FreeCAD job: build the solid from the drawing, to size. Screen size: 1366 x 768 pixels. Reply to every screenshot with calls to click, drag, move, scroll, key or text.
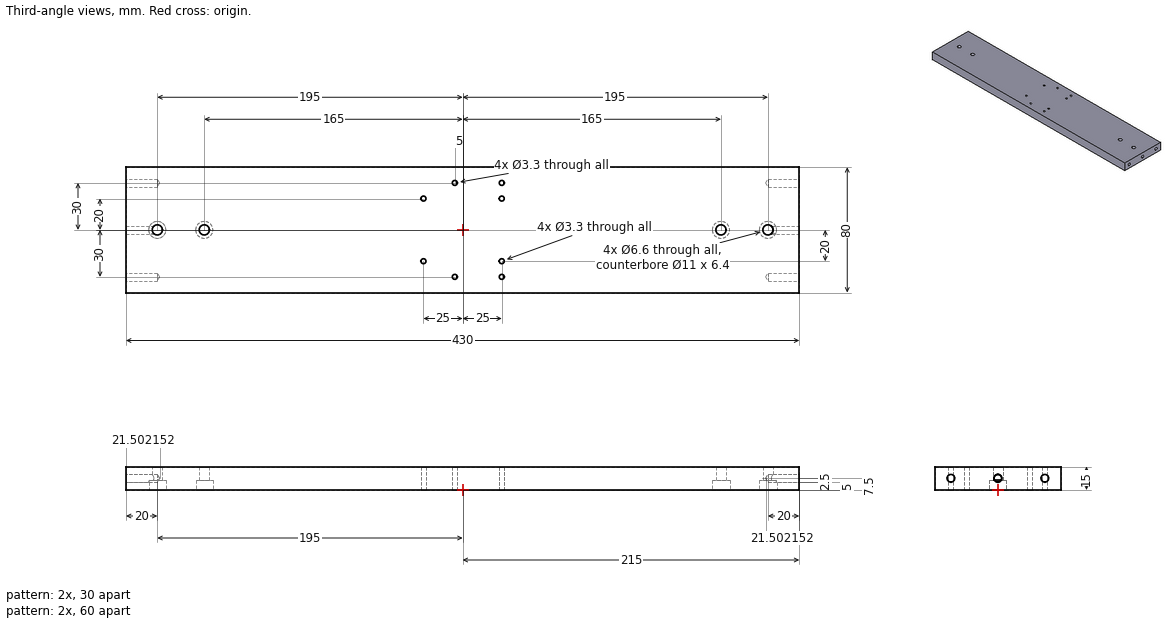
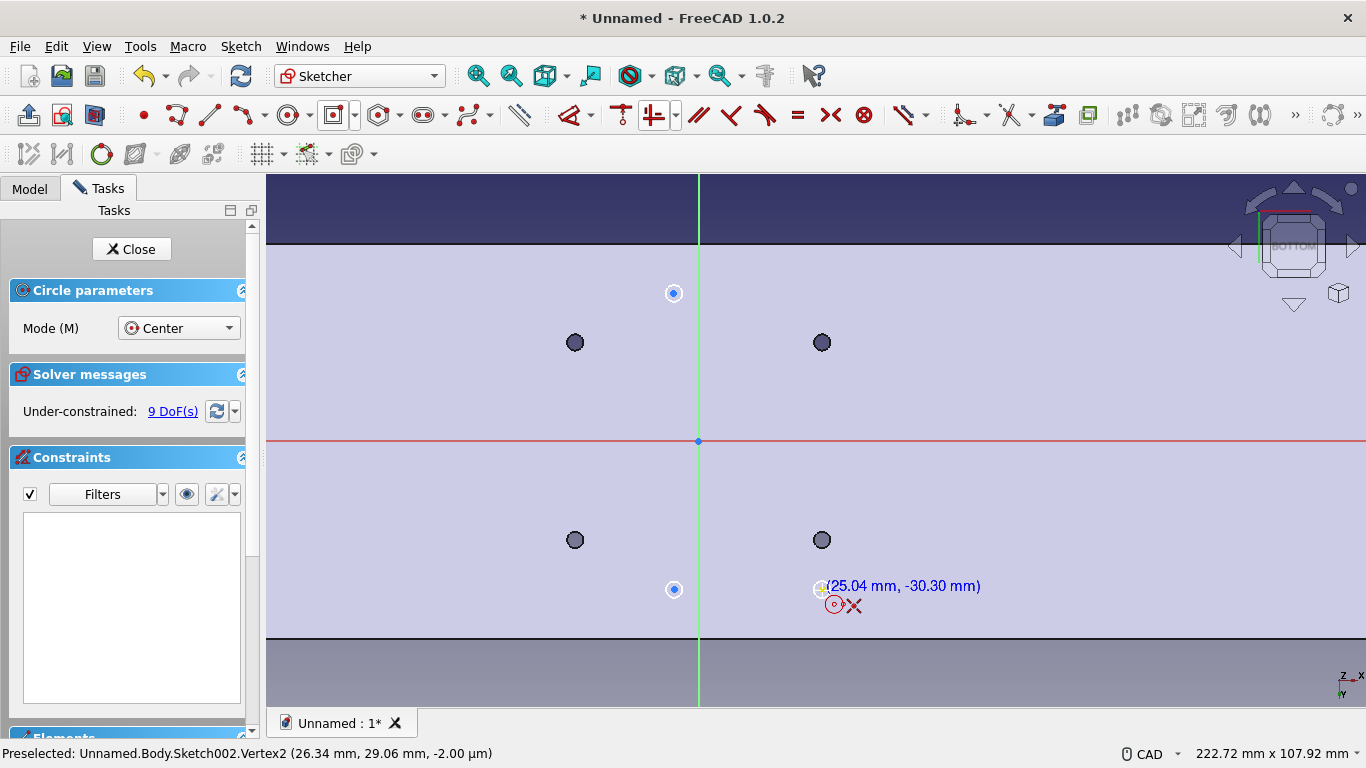
scroll(822, 293, up, 6)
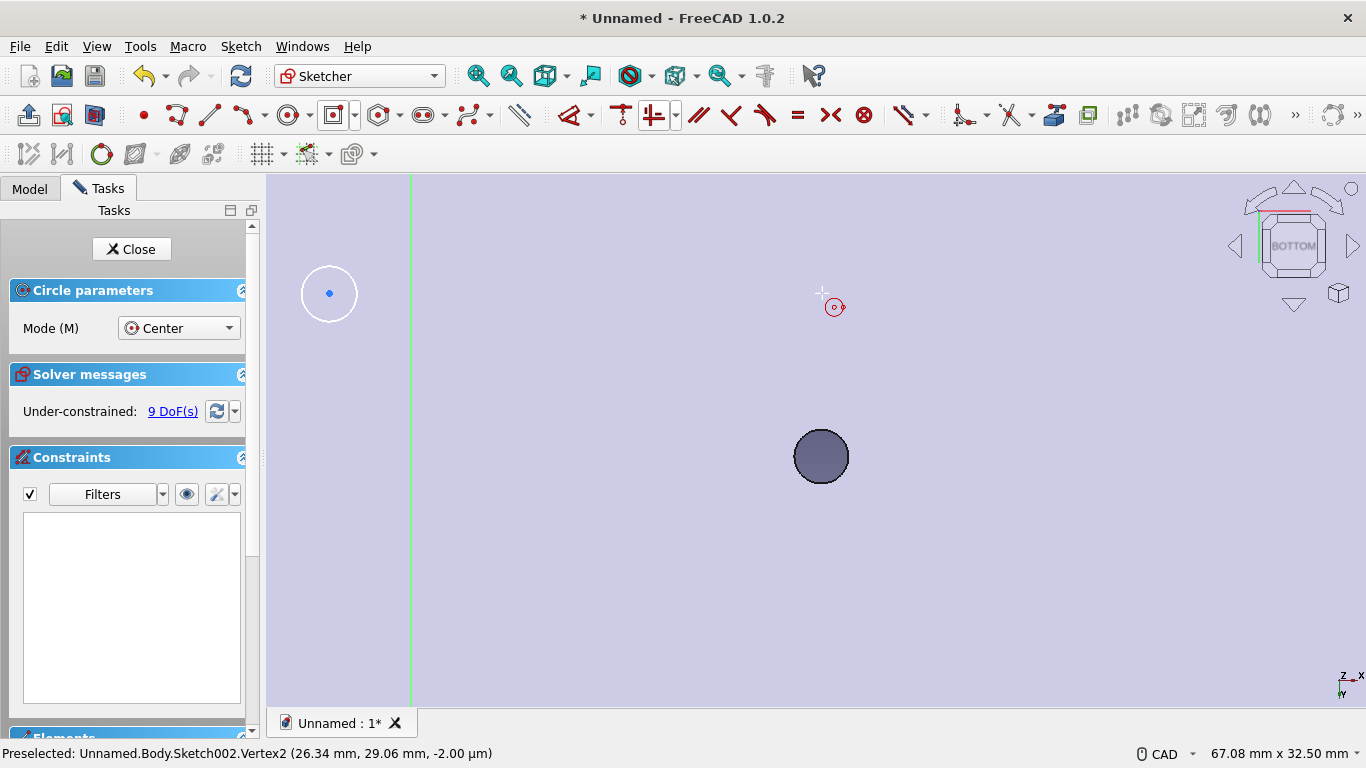
click(821, 293)
click(841, 273)
key(Escape)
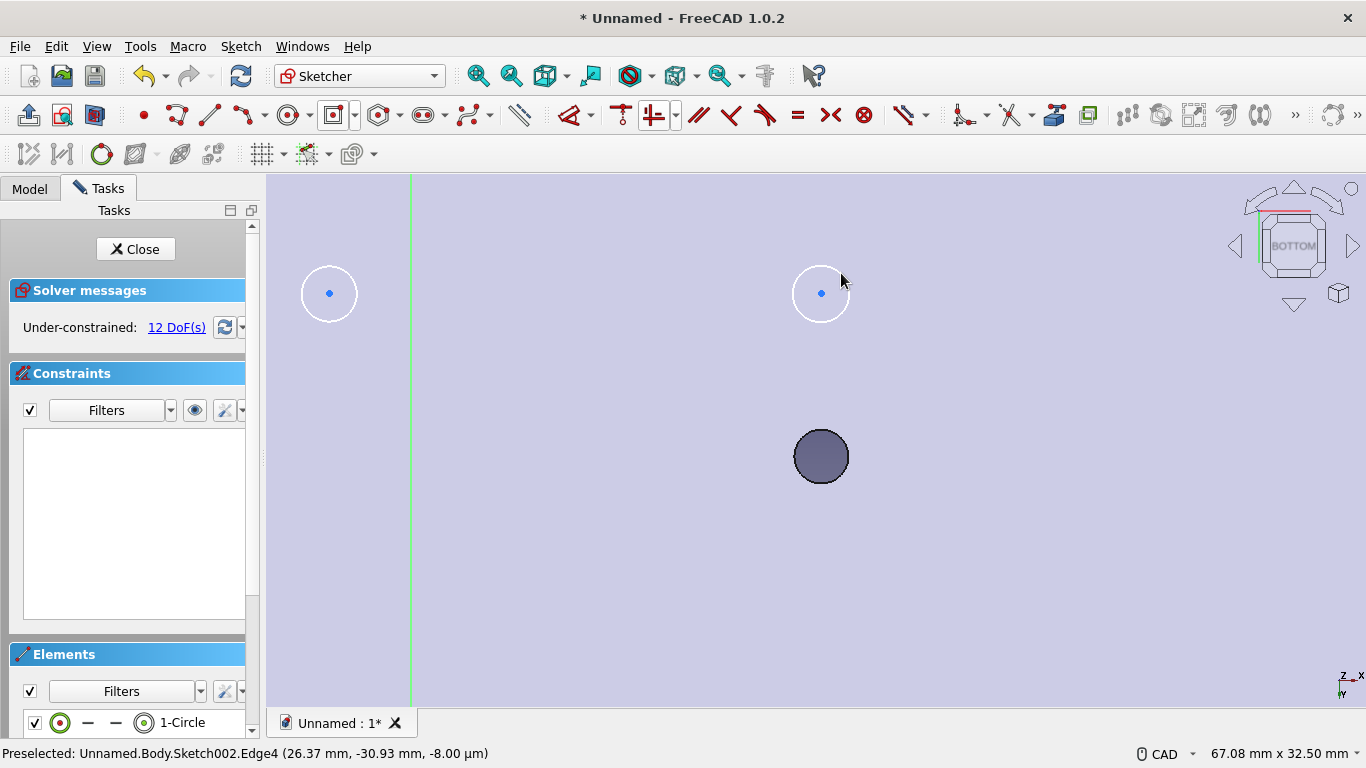
scroll(822, 292, down, 6)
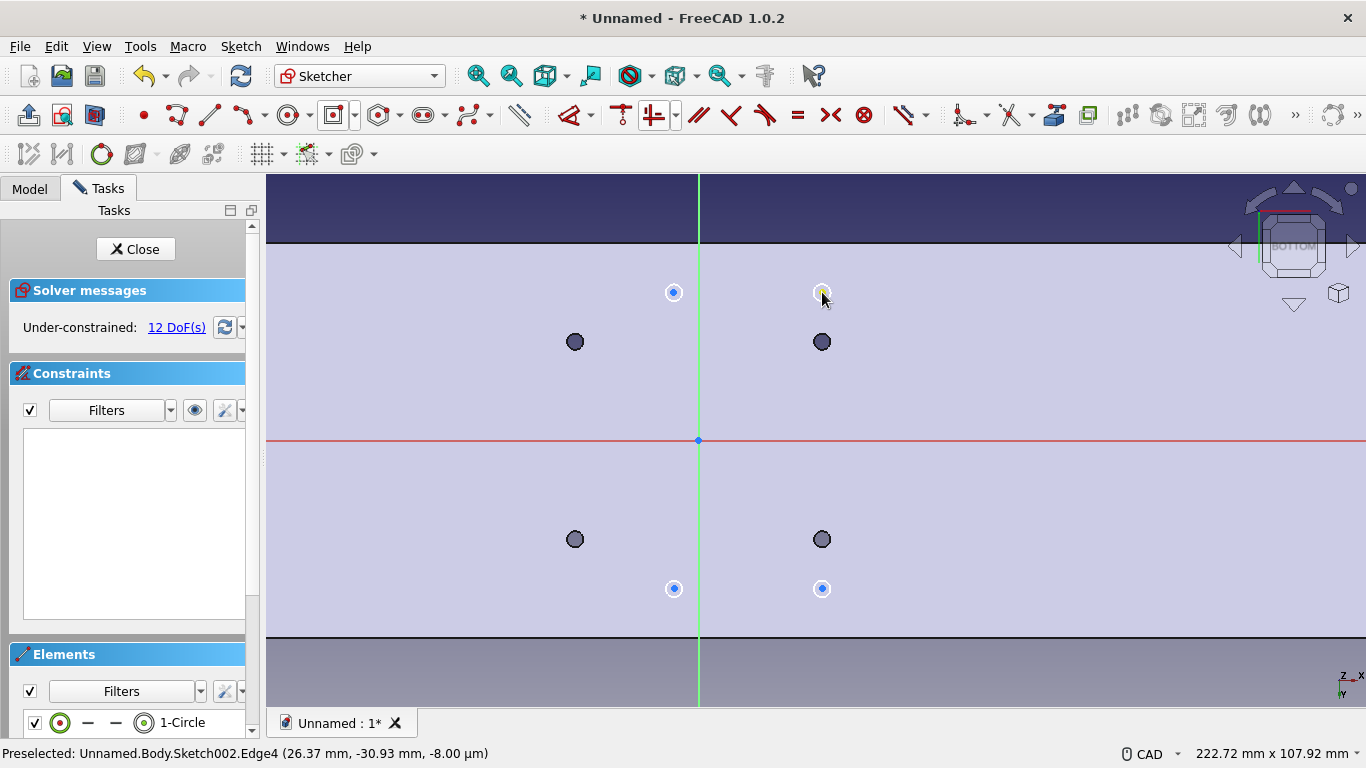
scroll(680, 583, up, 3)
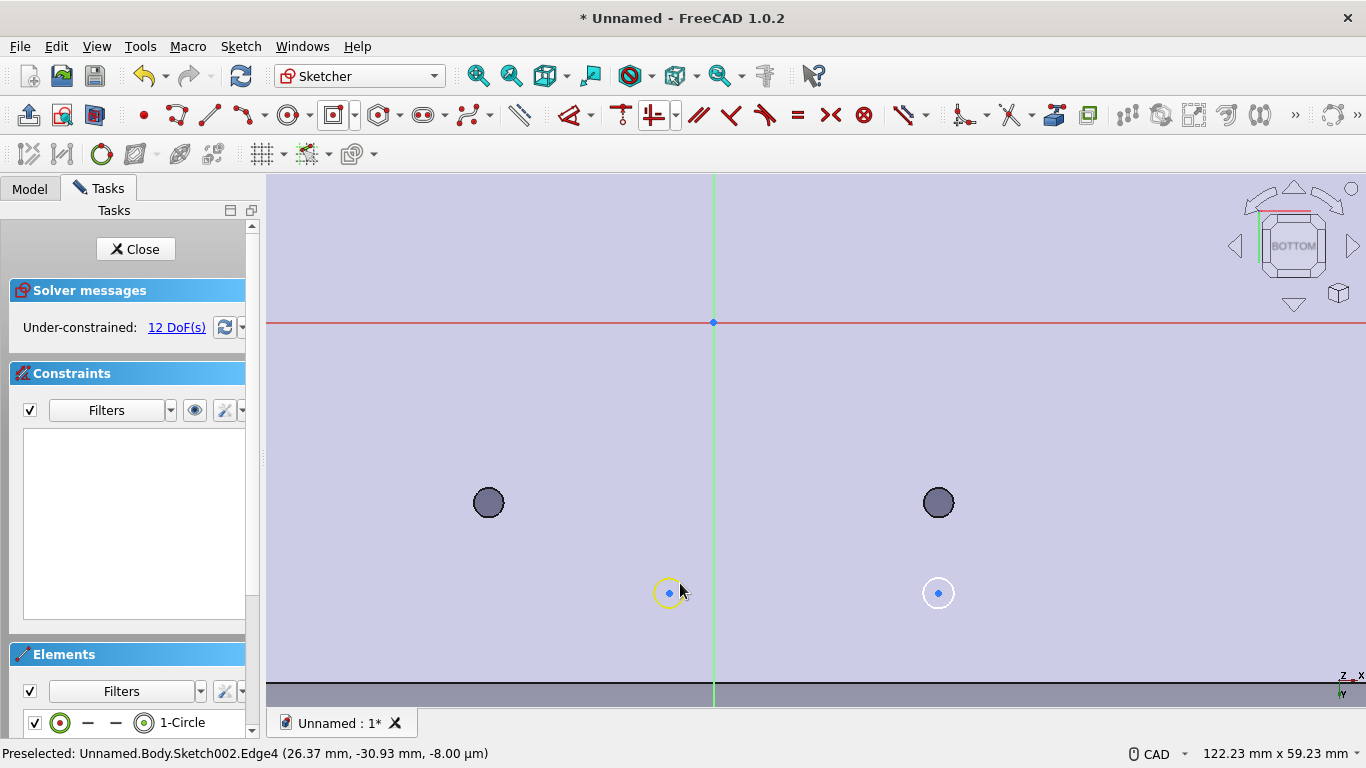
click(679, 583)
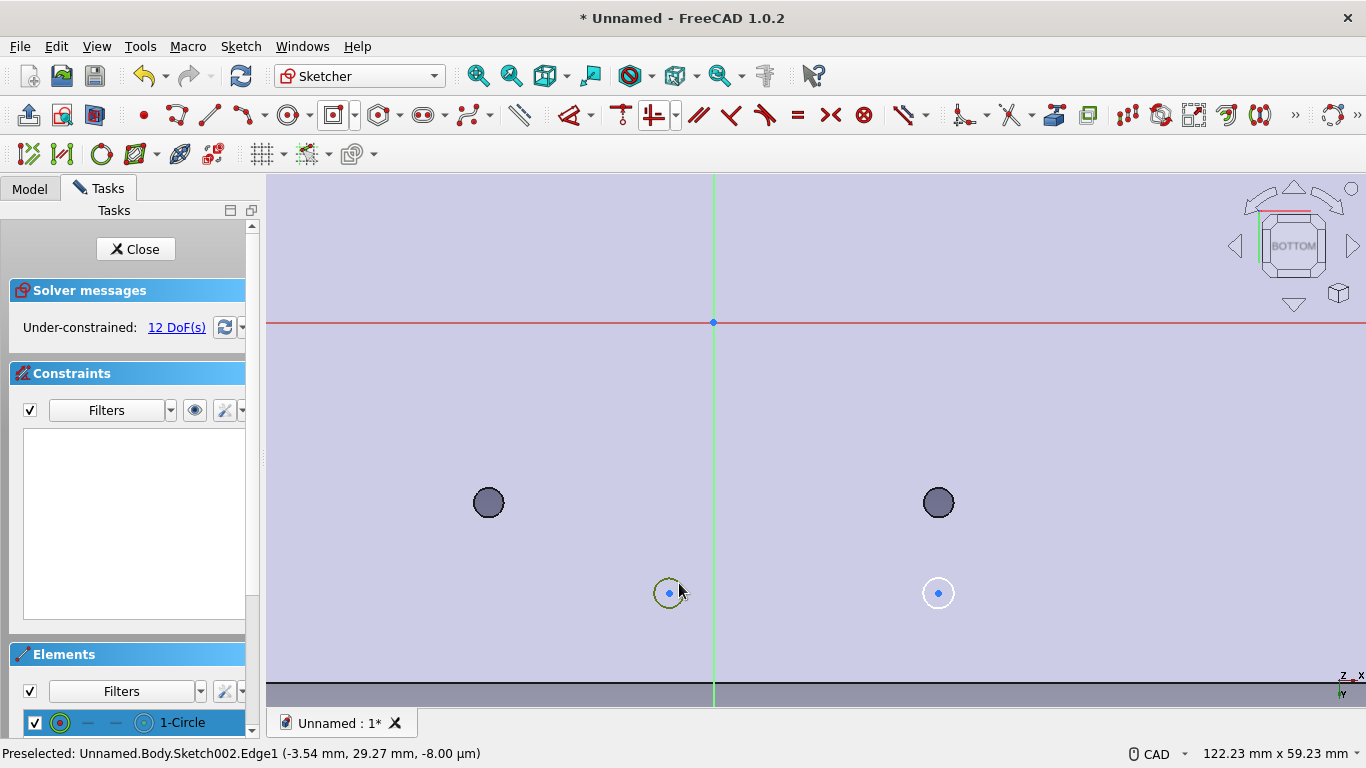
scroll(679, 584, down, 3)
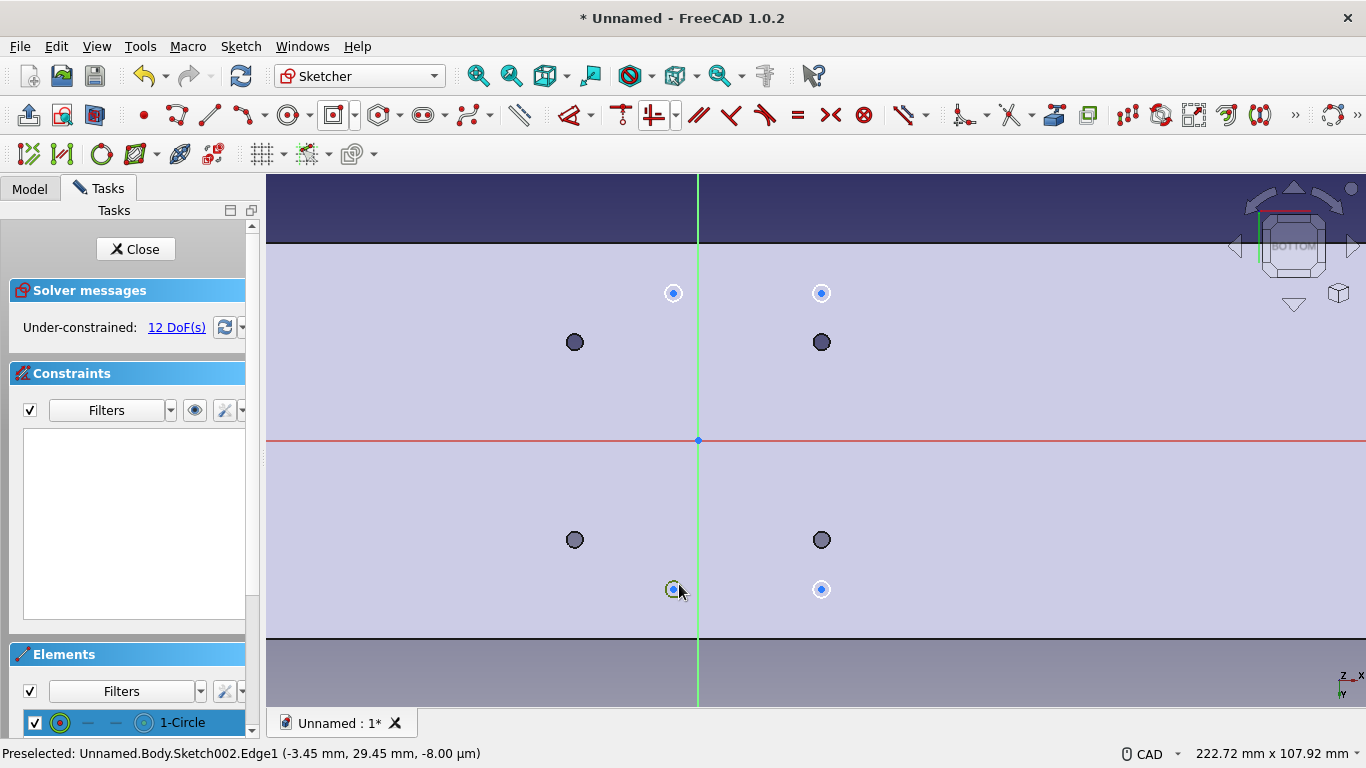
scroll(679, 287, up, 3)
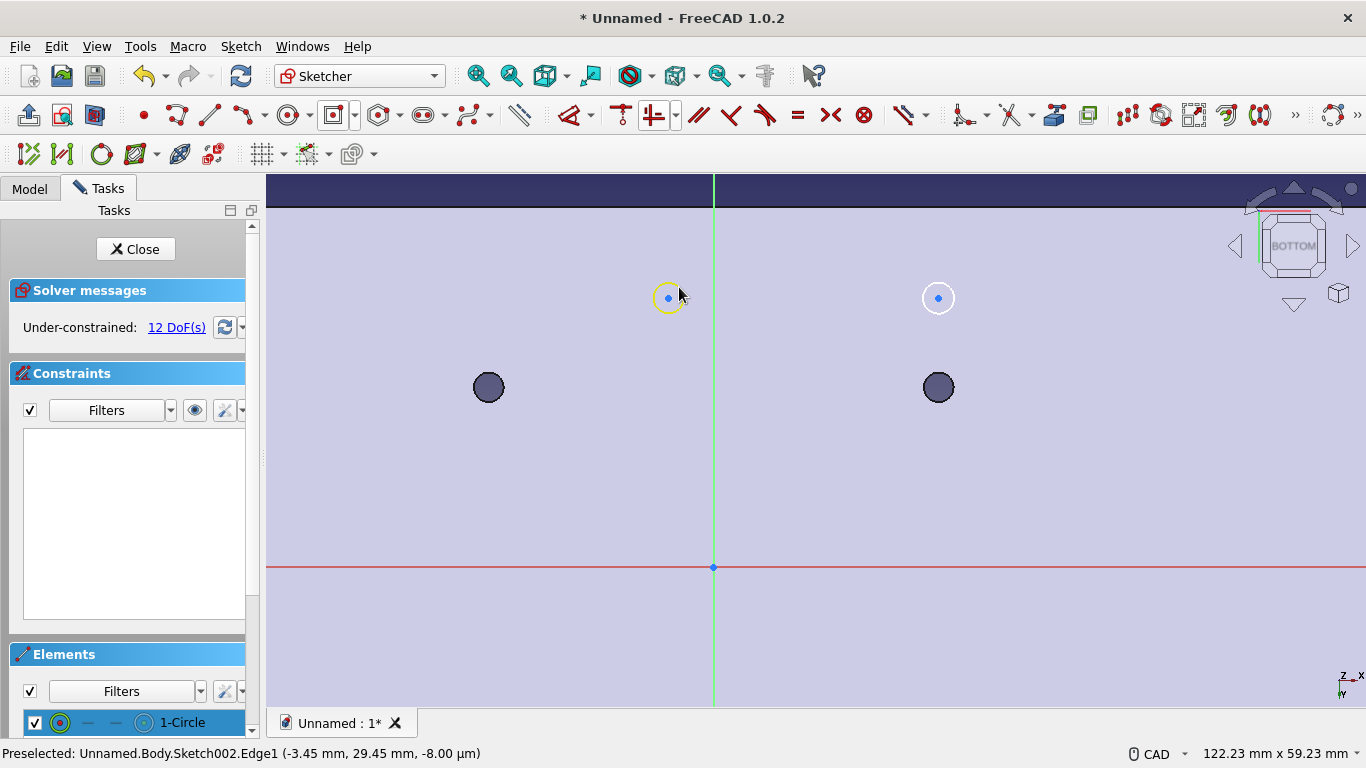
click(679, 287)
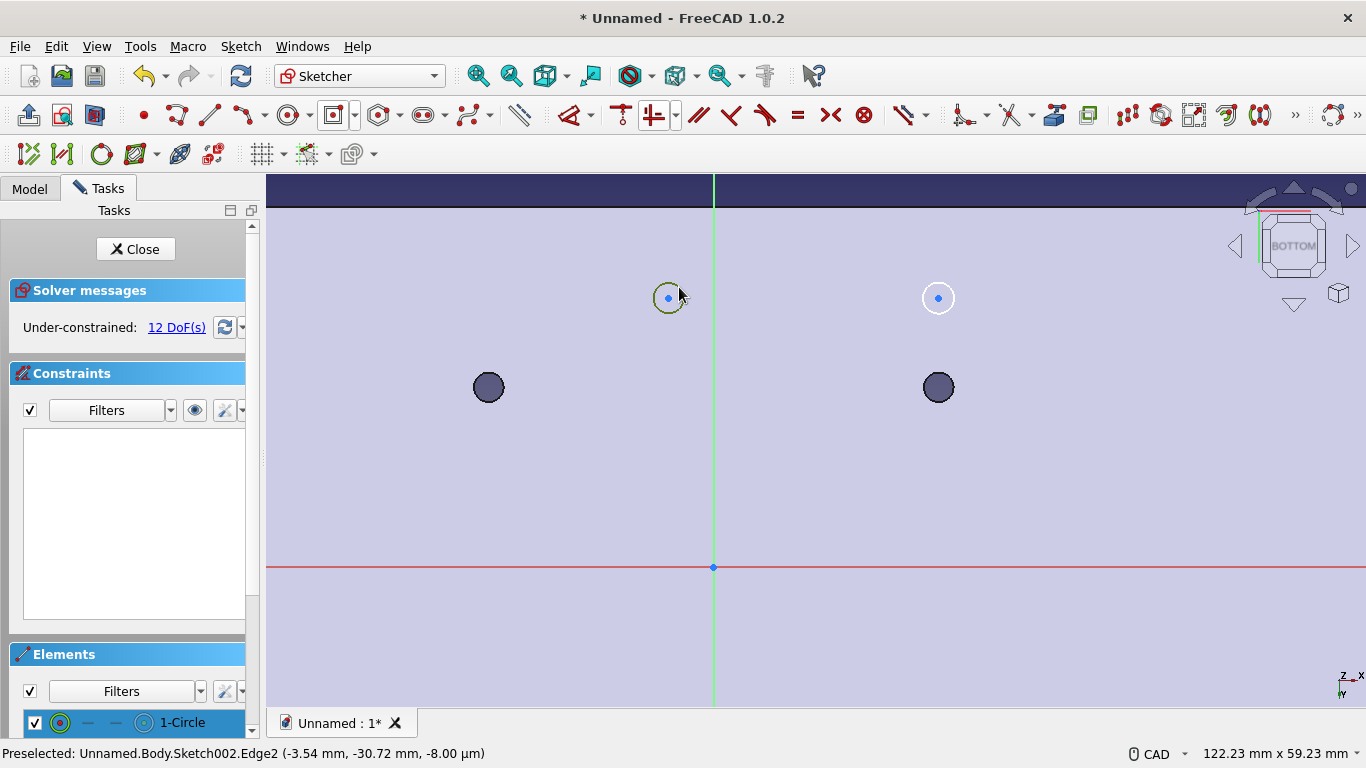
scroll(679, 286, down, 3)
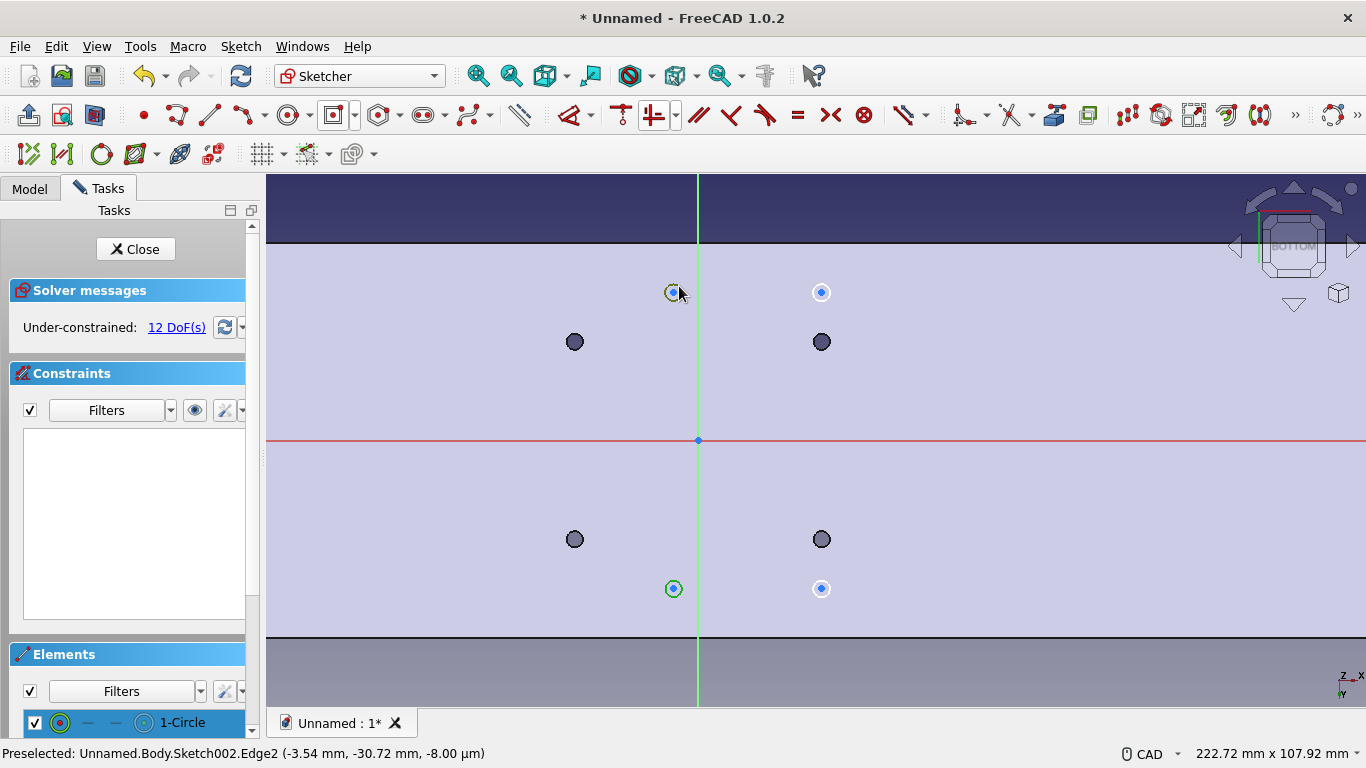
scroll(827, 583, up, 3)